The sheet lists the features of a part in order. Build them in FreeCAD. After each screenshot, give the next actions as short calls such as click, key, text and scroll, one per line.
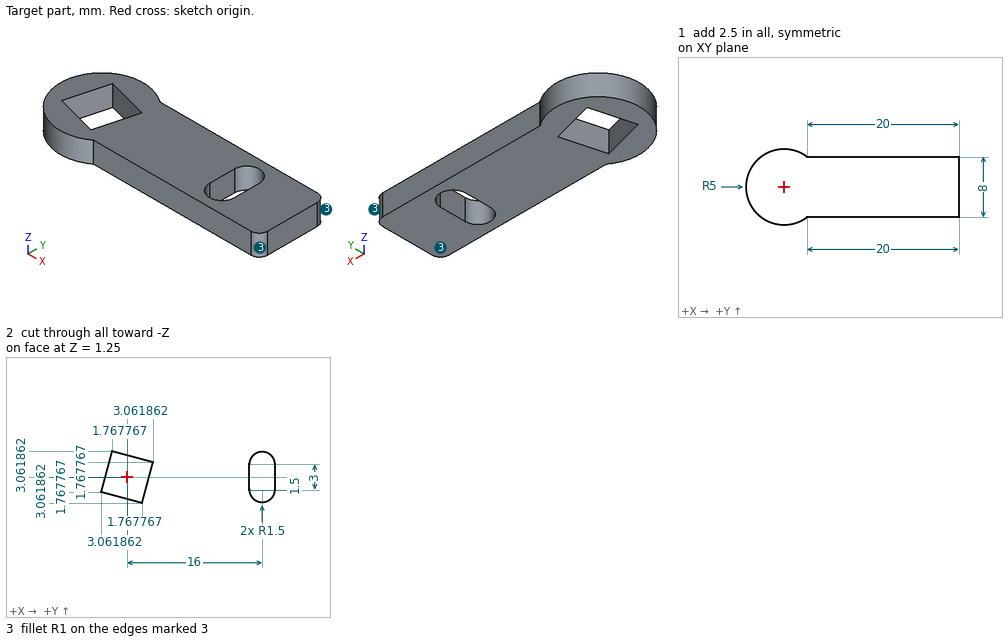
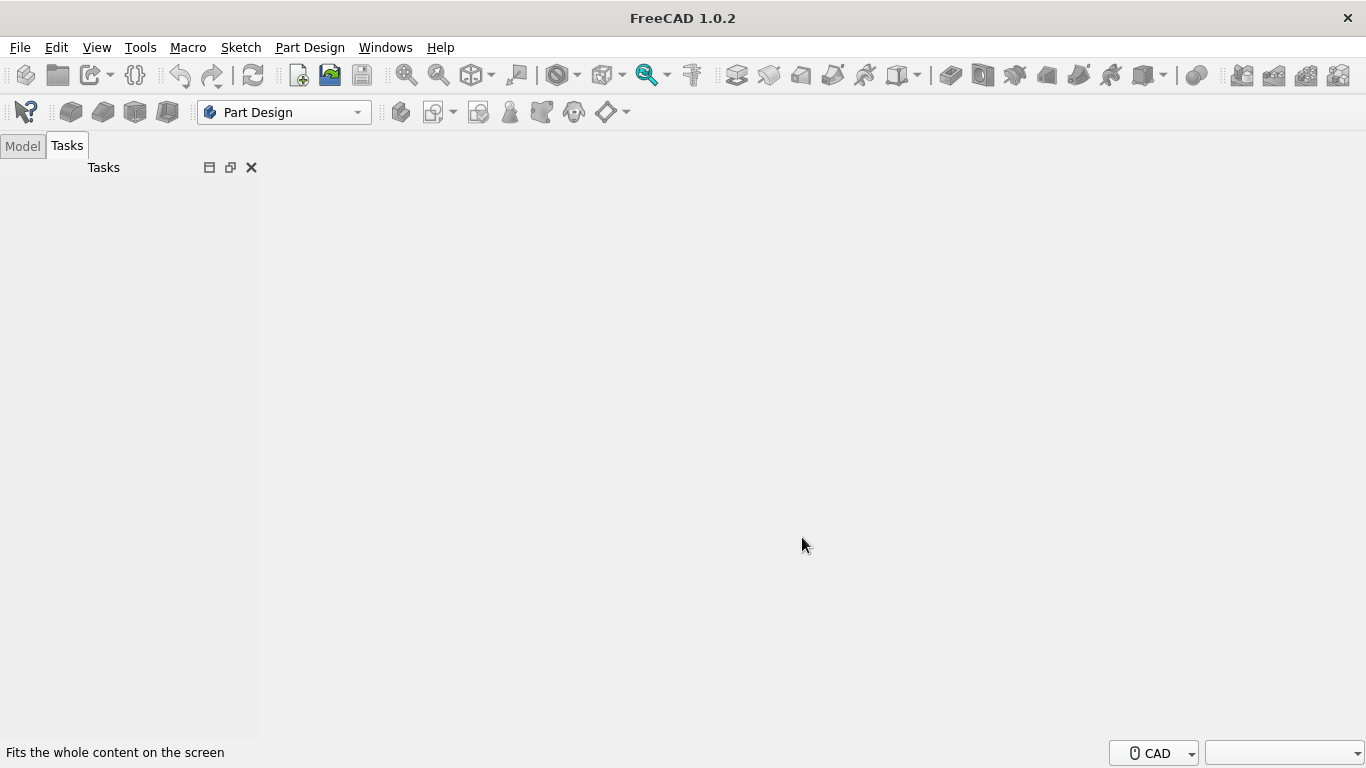
key(ctrl+n)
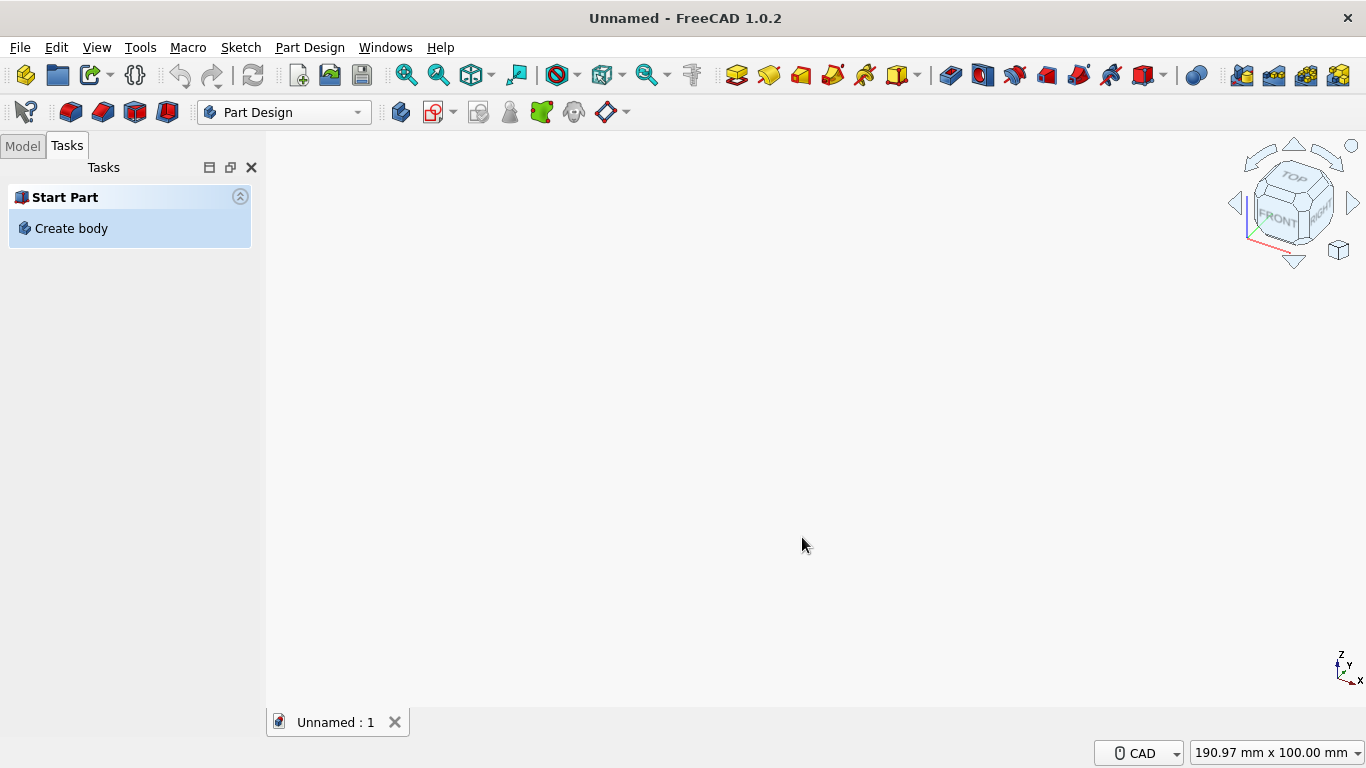
click(434, 112)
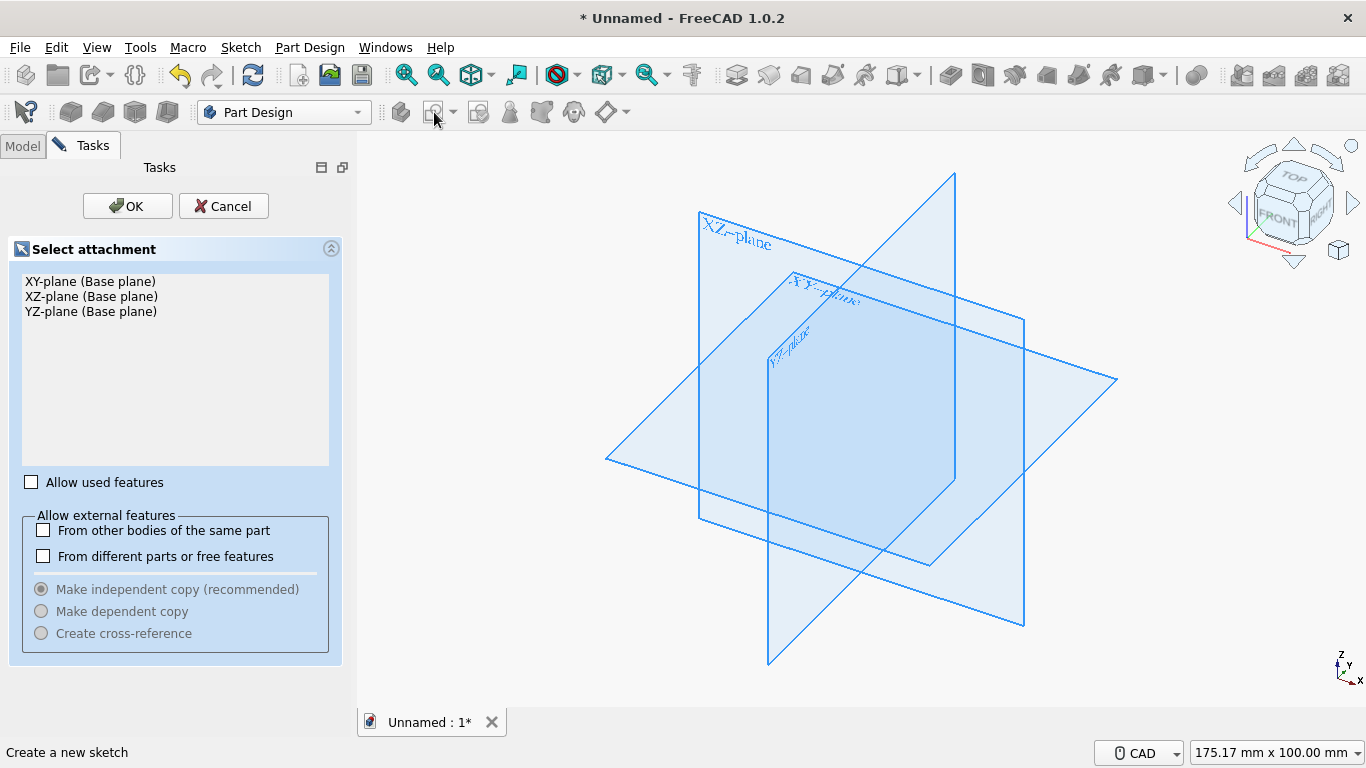
click(82, 282)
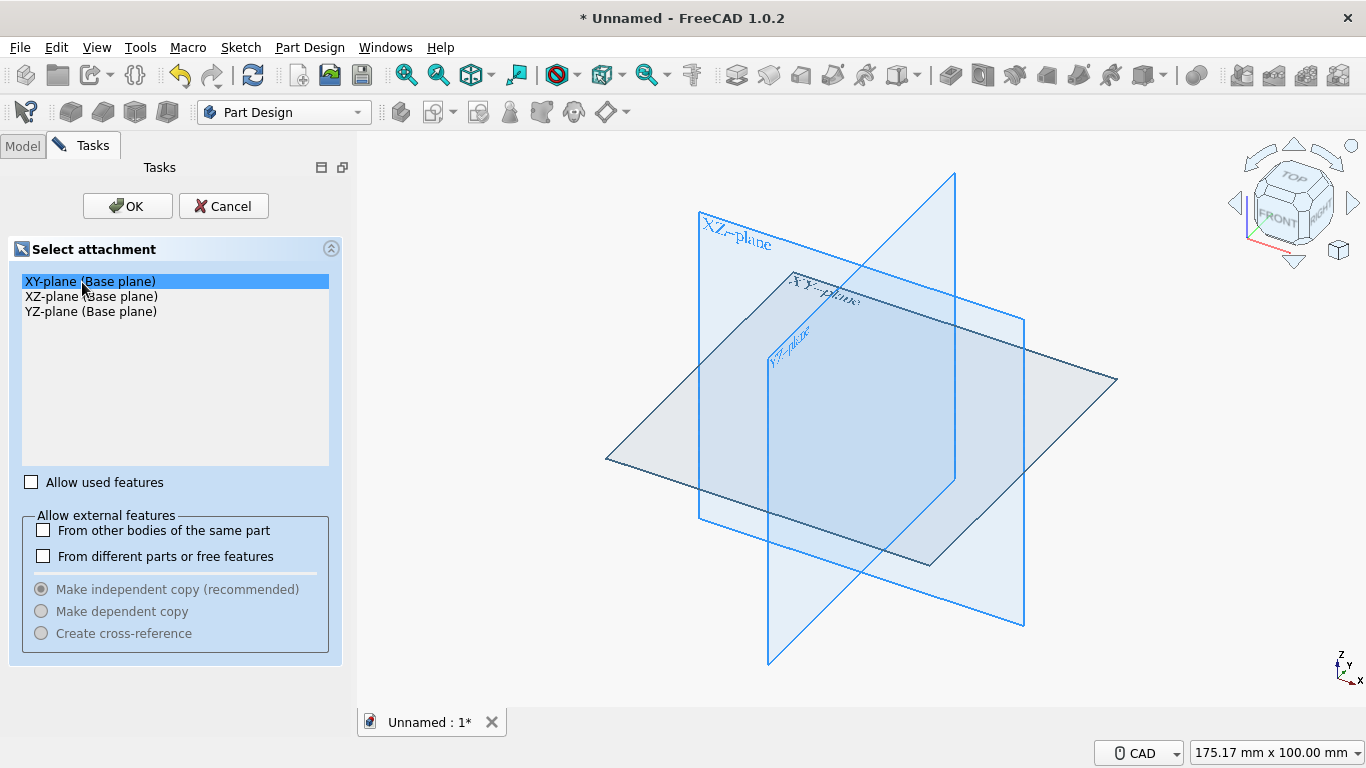
click(128, 206)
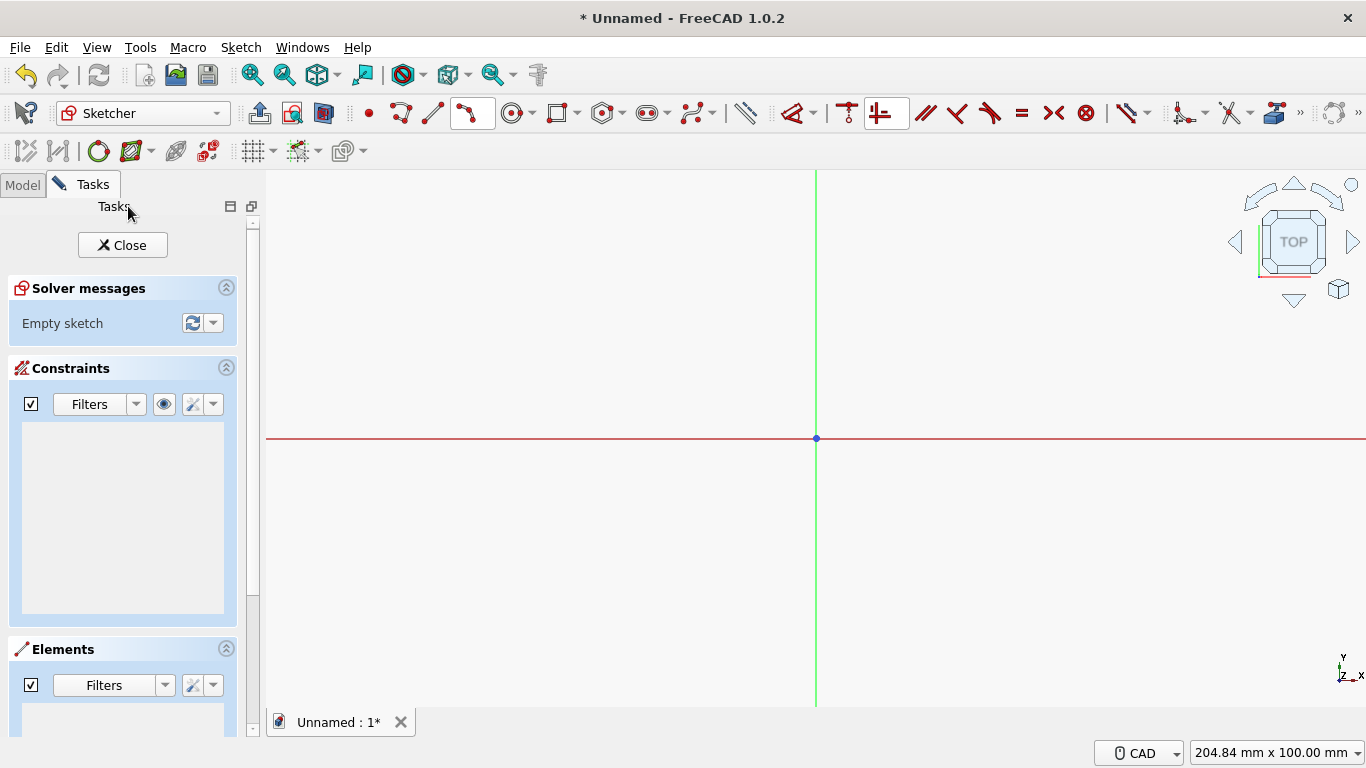
scroll(903, 438, up, 7)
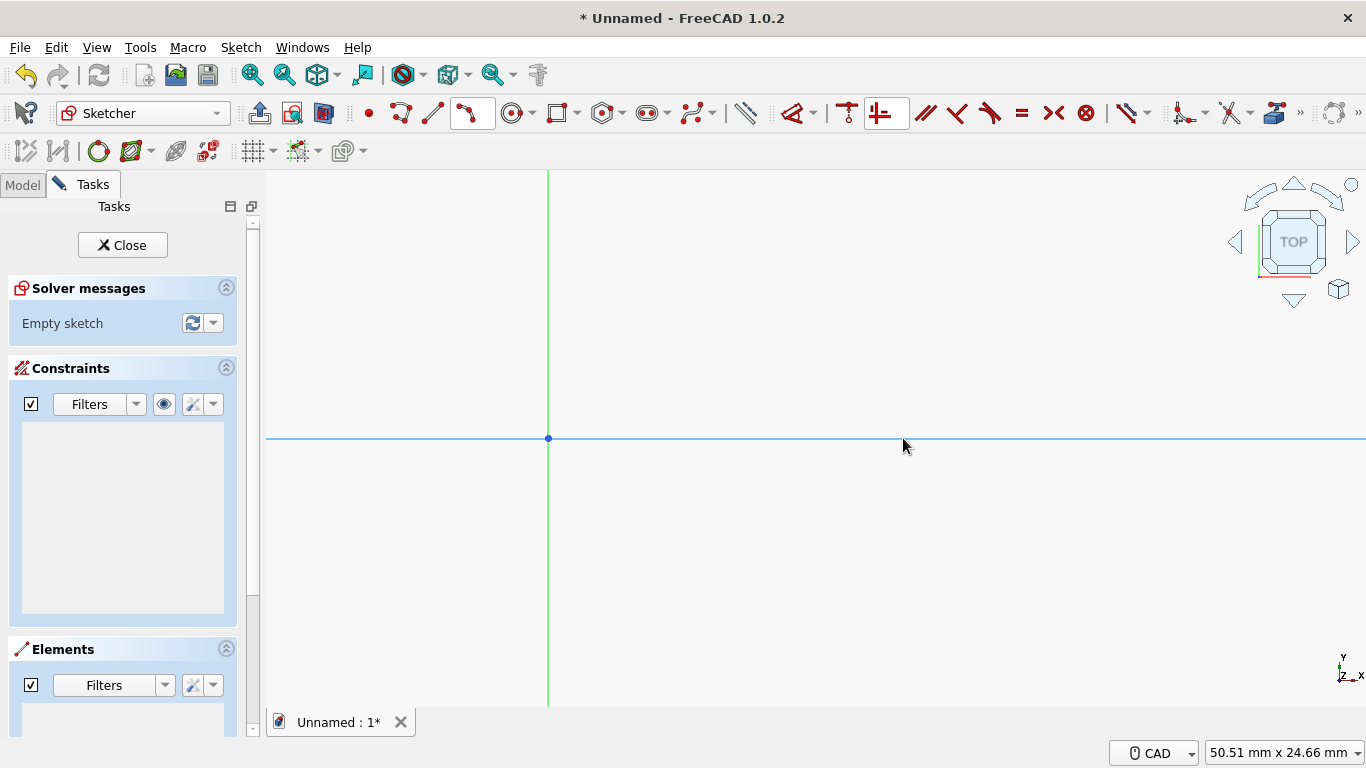
click(402, 114)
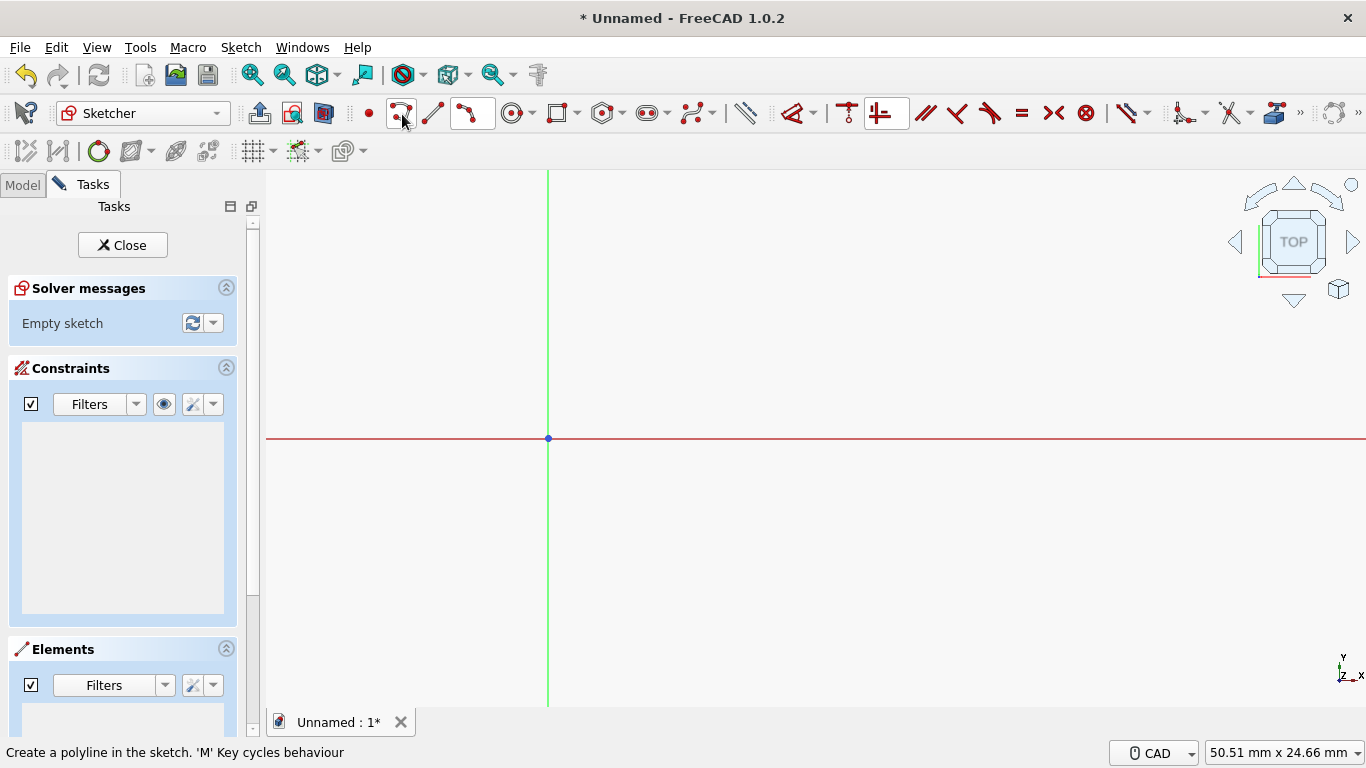
click(614, 526)
click(1049, 526)
click(1049, 351)
click(614, 351)
right_click(614, 351)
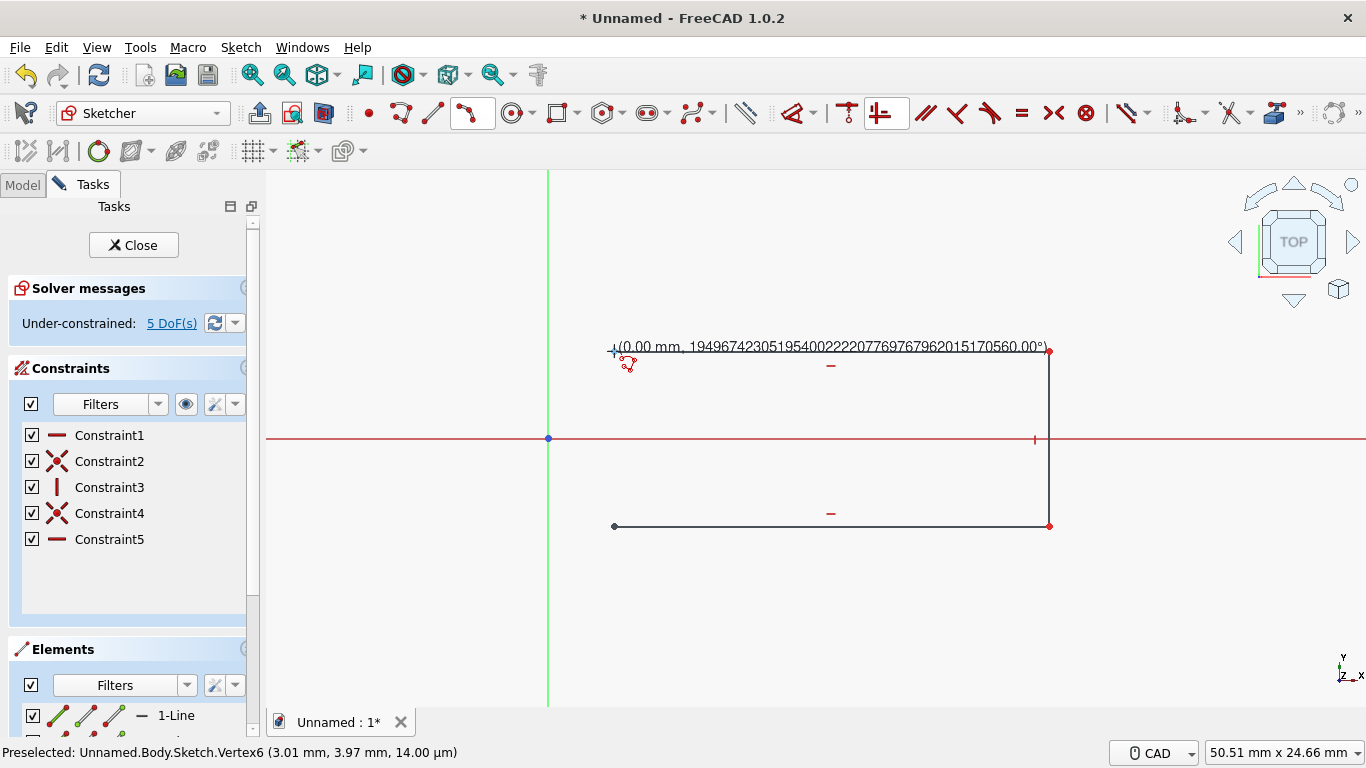
key(g)
key(3)
key(a)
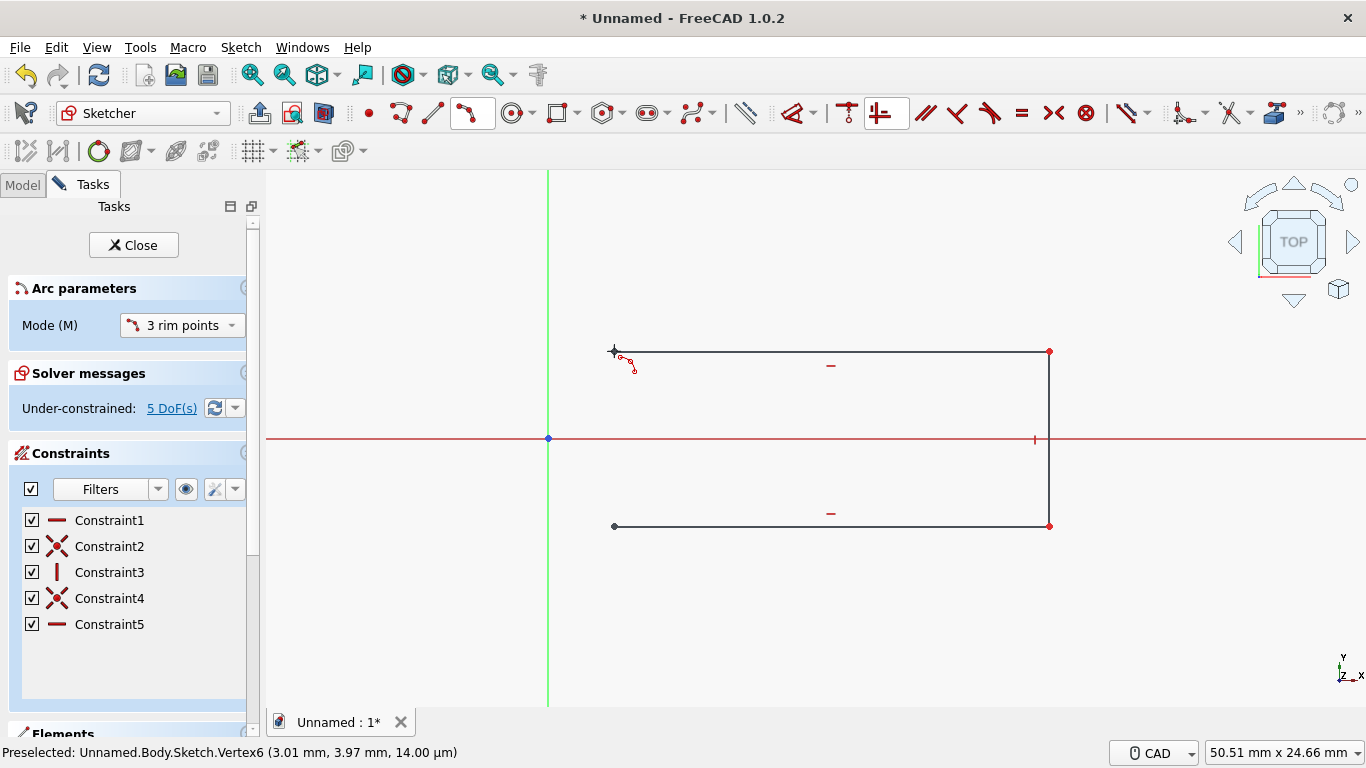
click(614, 352)
click(614, 527)
click(450, 392)
key(Escape)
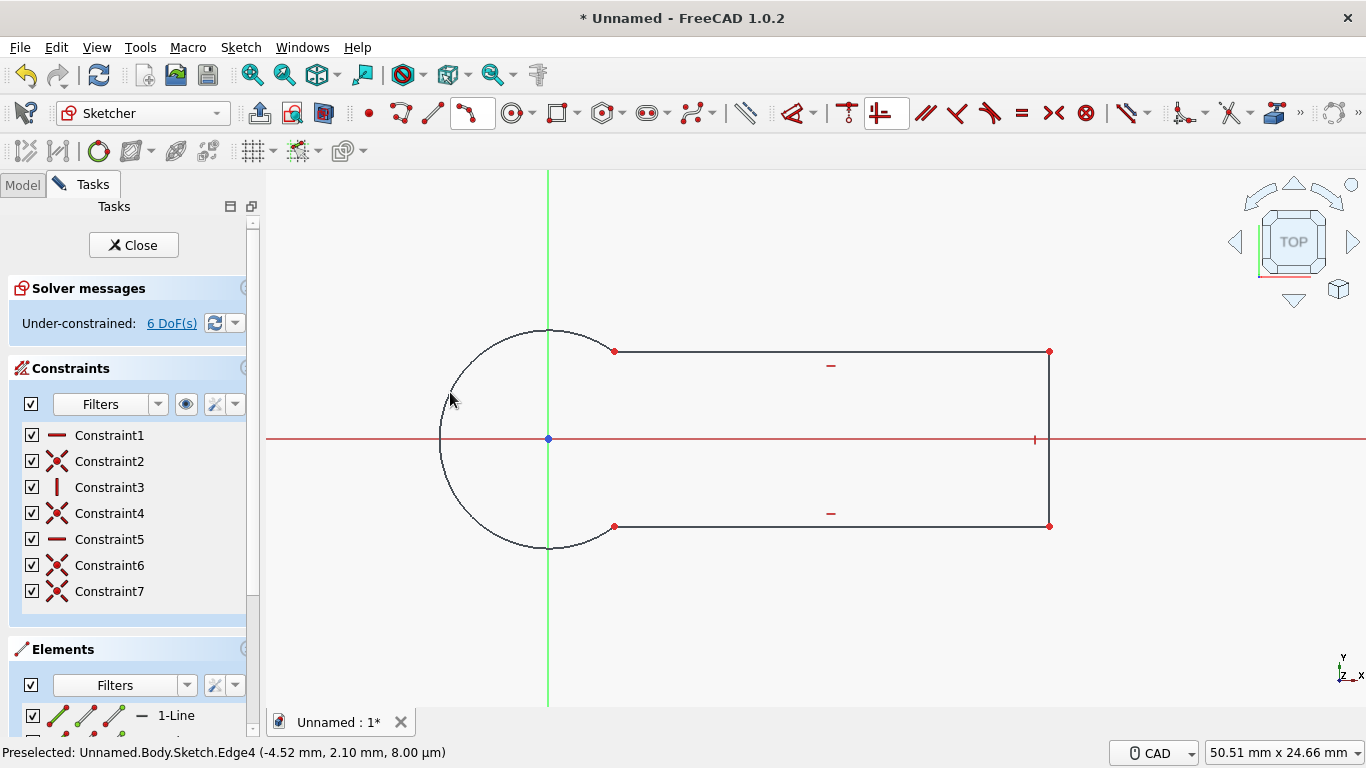
drag(538, 428, 559, 449)